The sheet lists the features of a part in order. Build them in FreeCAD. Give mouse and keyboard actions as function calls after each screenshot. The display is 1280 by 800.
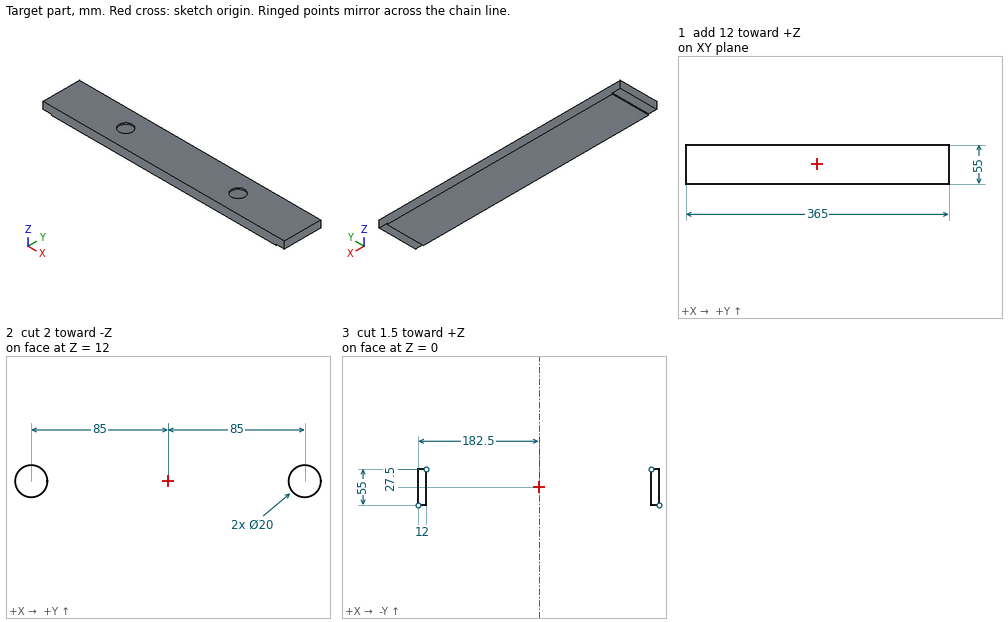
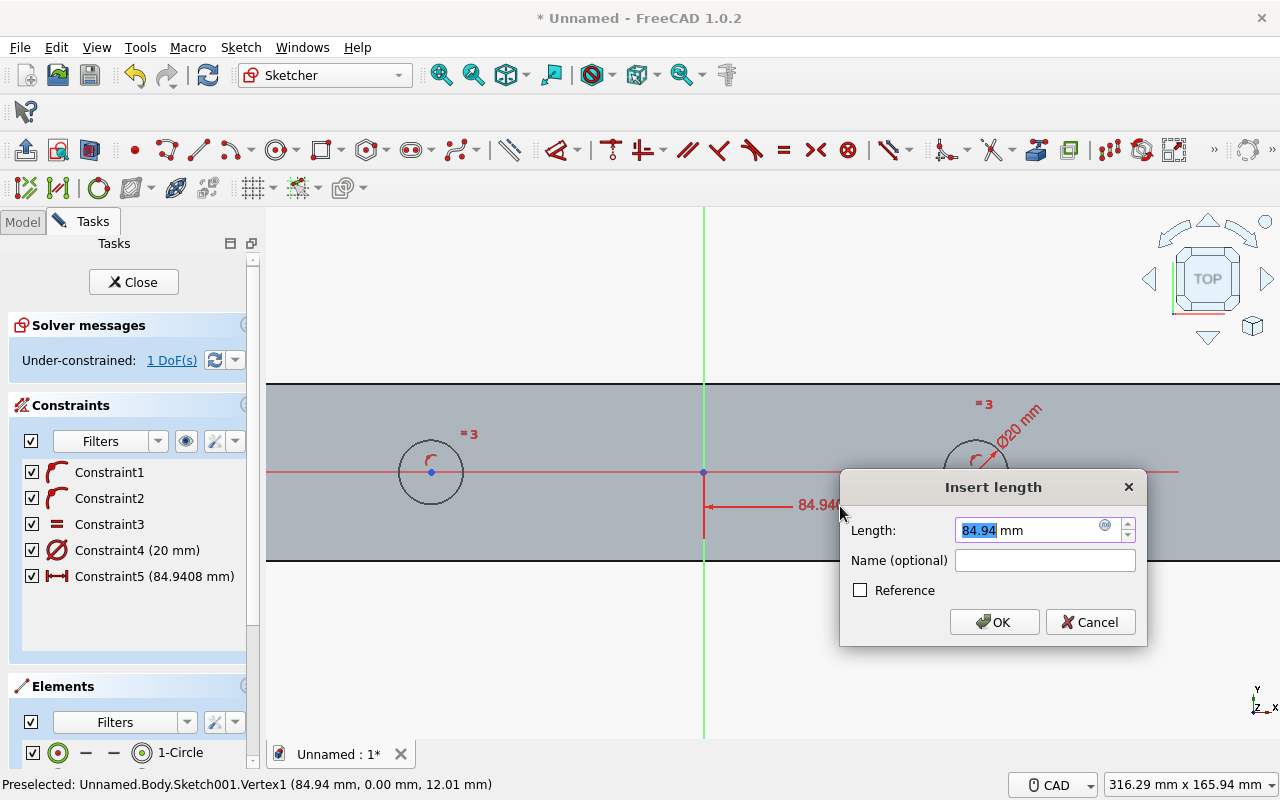
text(85)
key(Return)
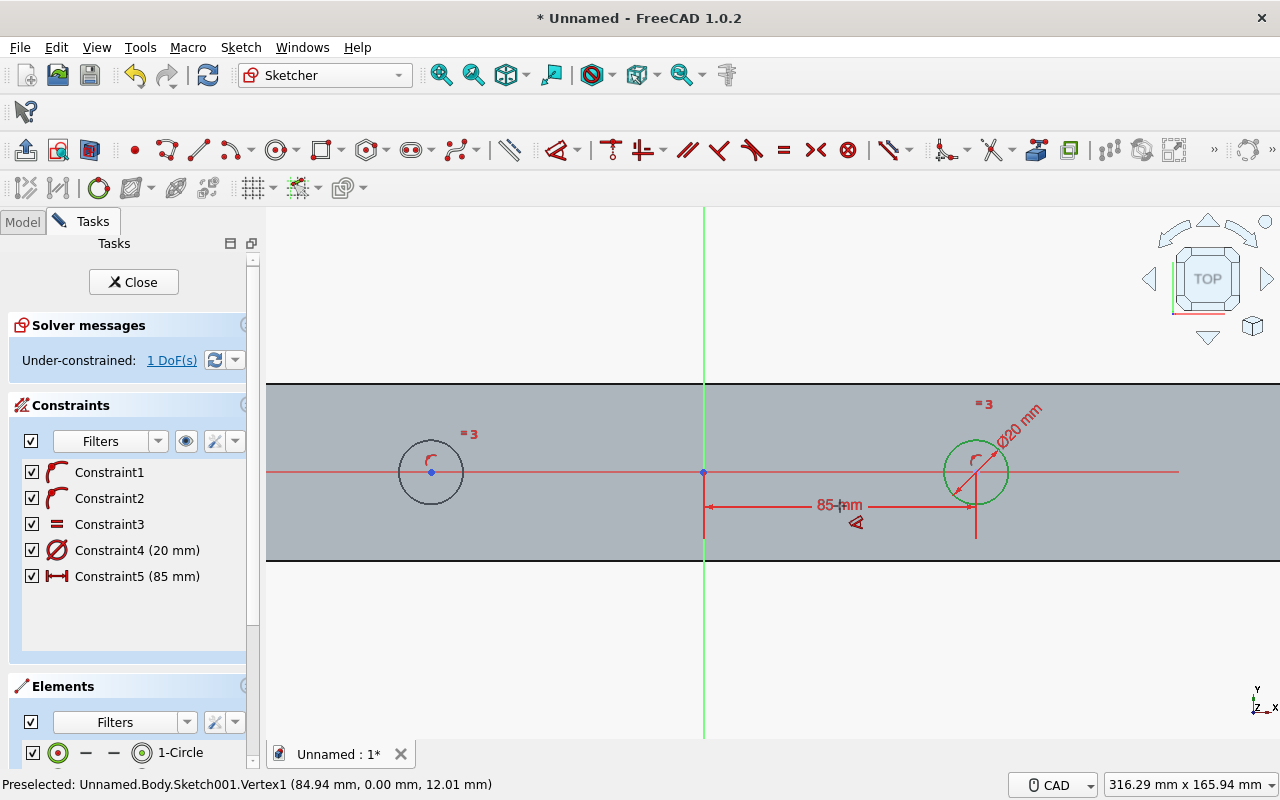
click(431, 472)
click(567, 506)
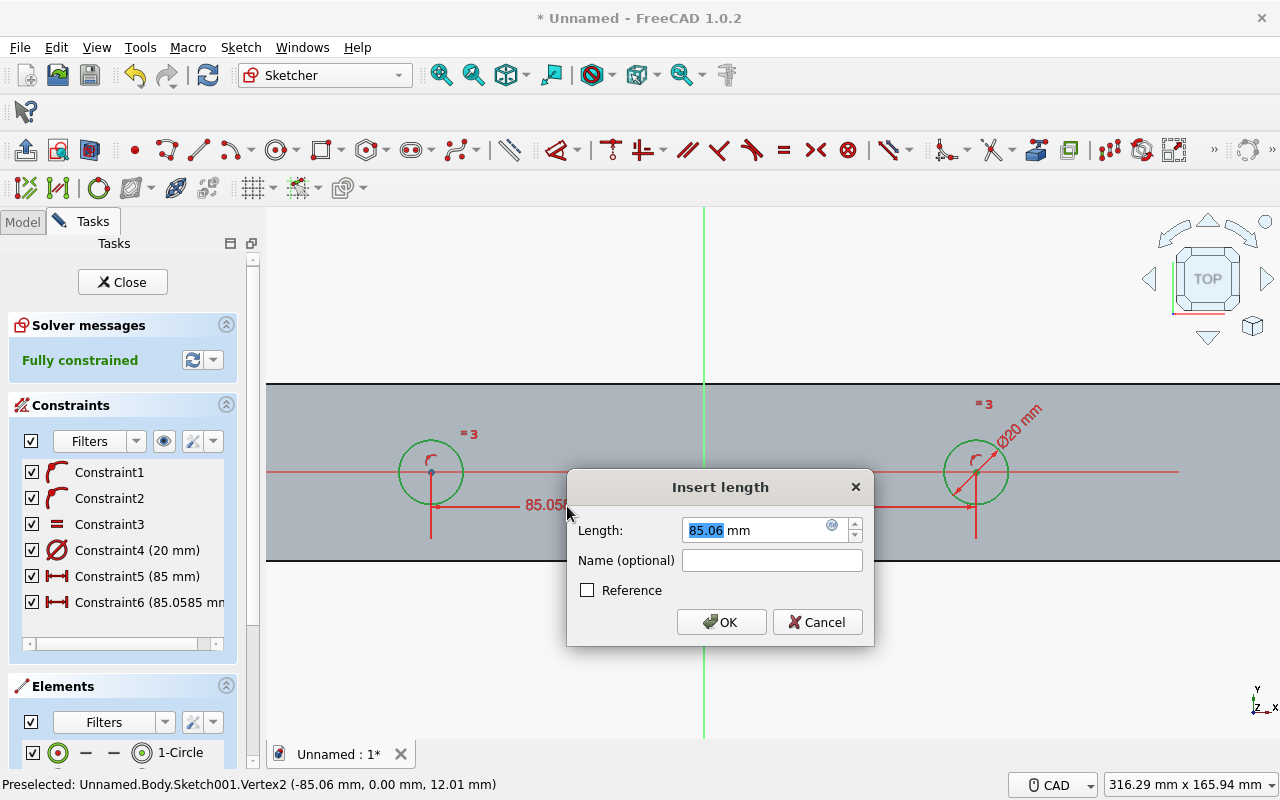
text(85)
key(Return)
key(Escape)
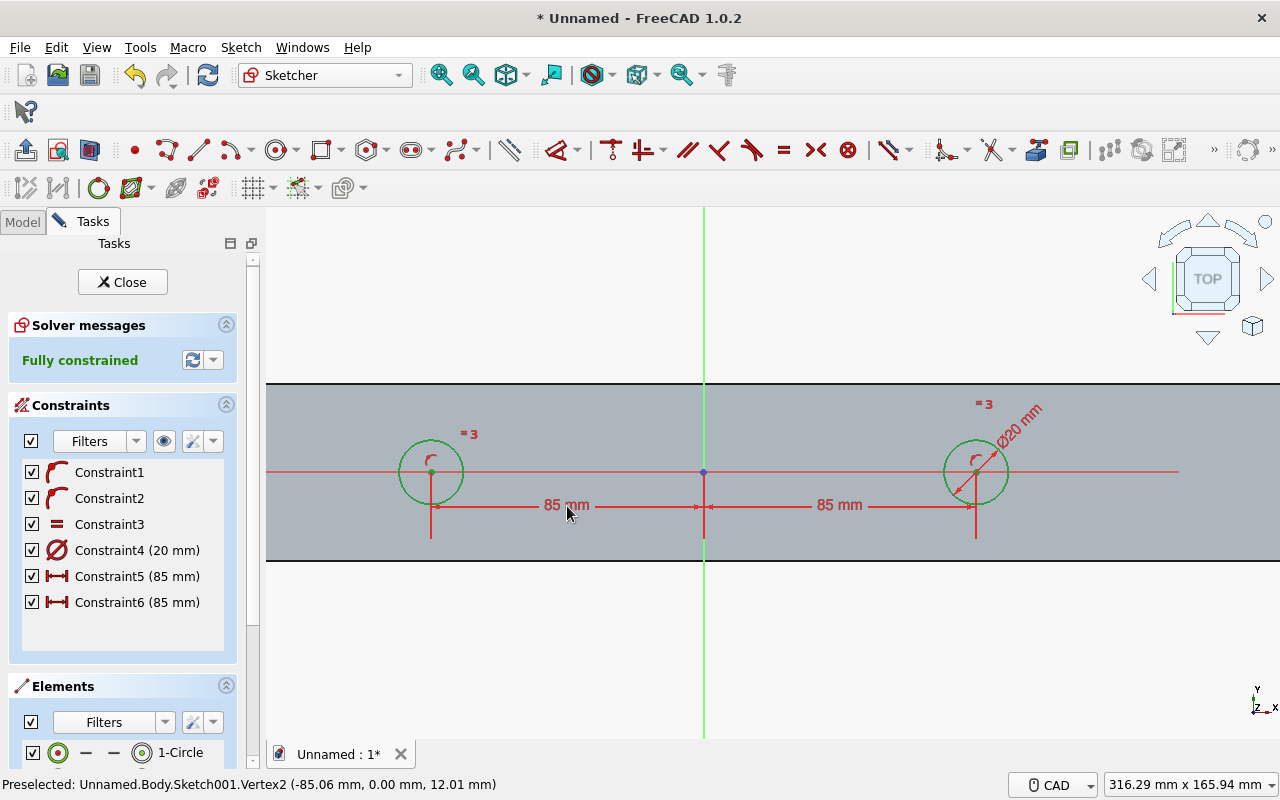
click(123, 282)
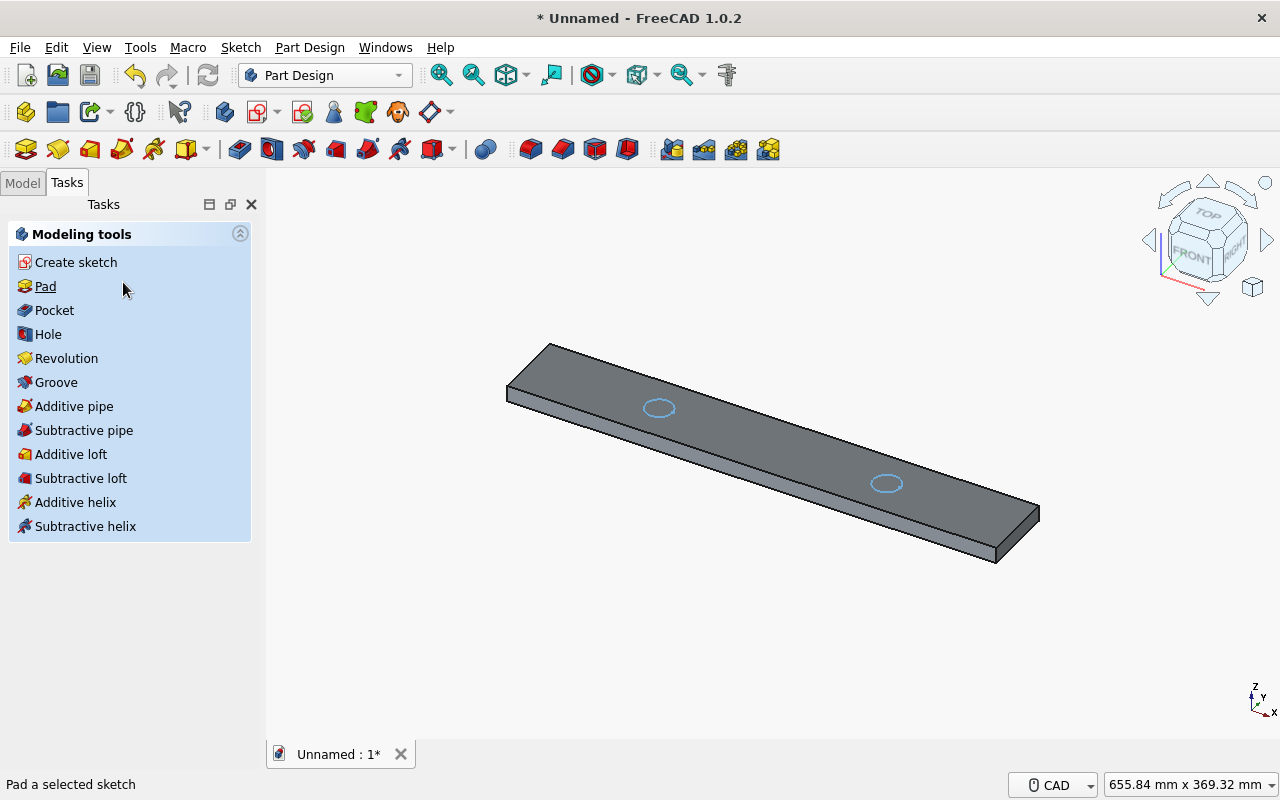
click(240, 150)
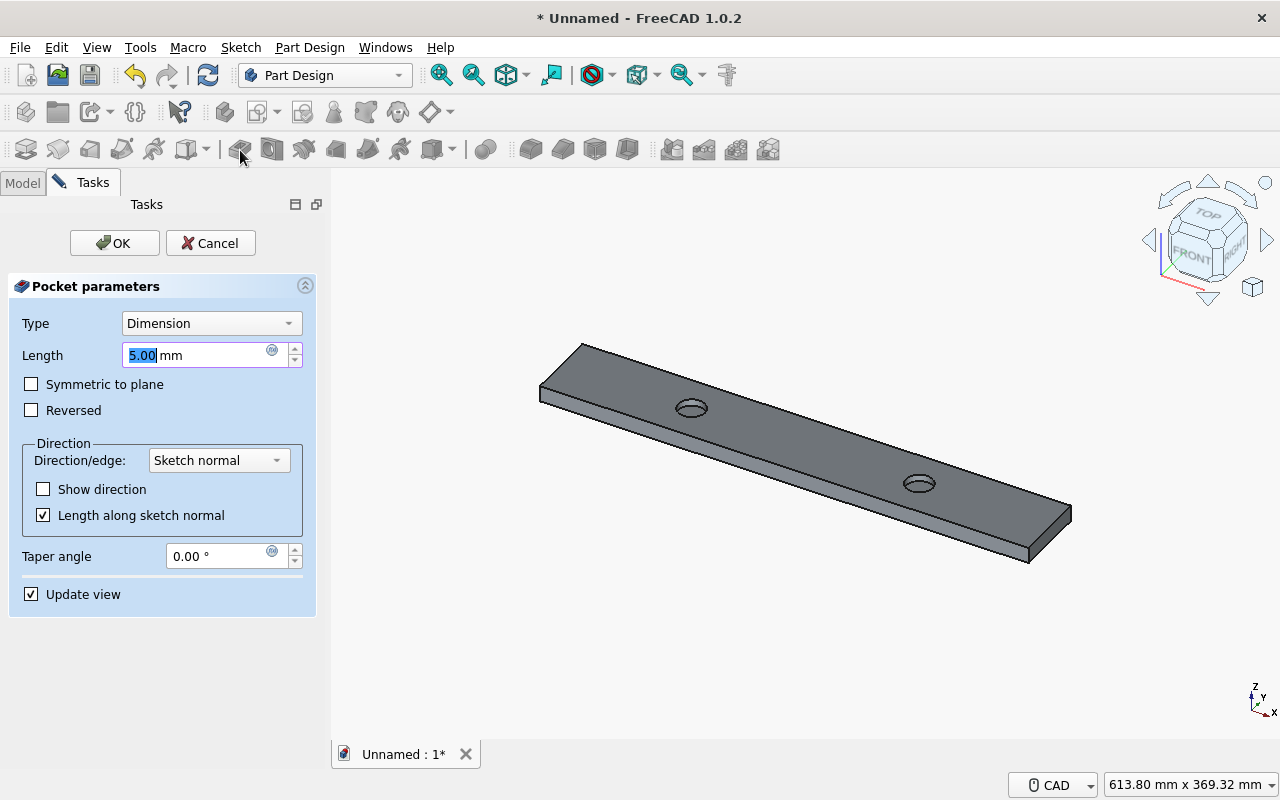
text(2)
key(Tab)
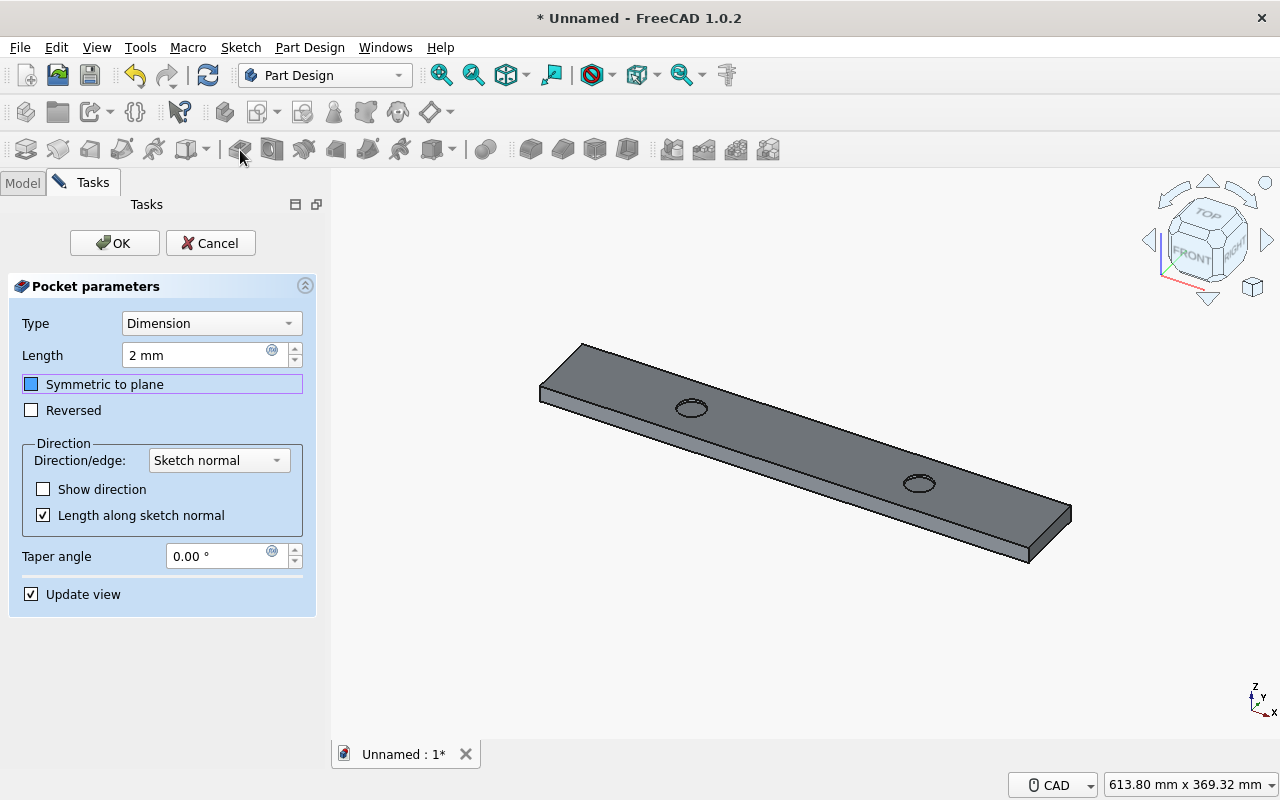
click(115, 243)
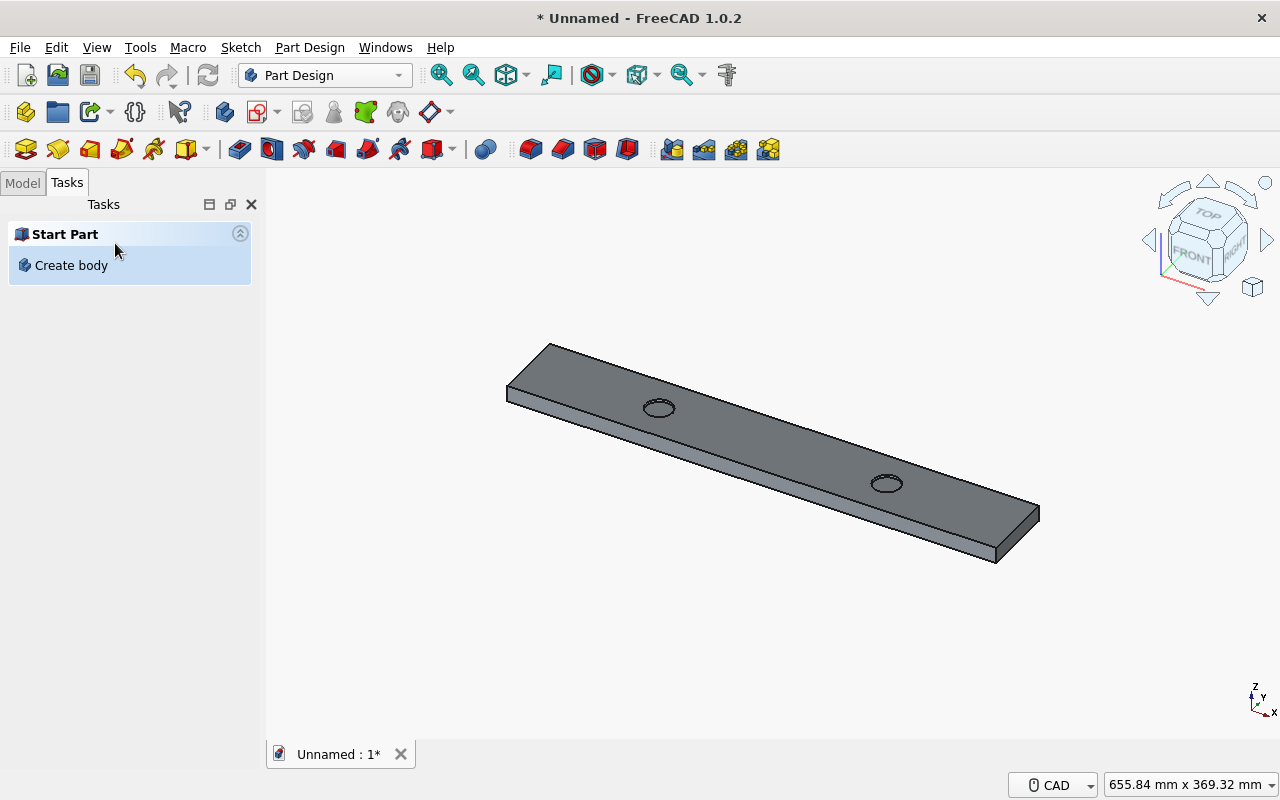
key(5)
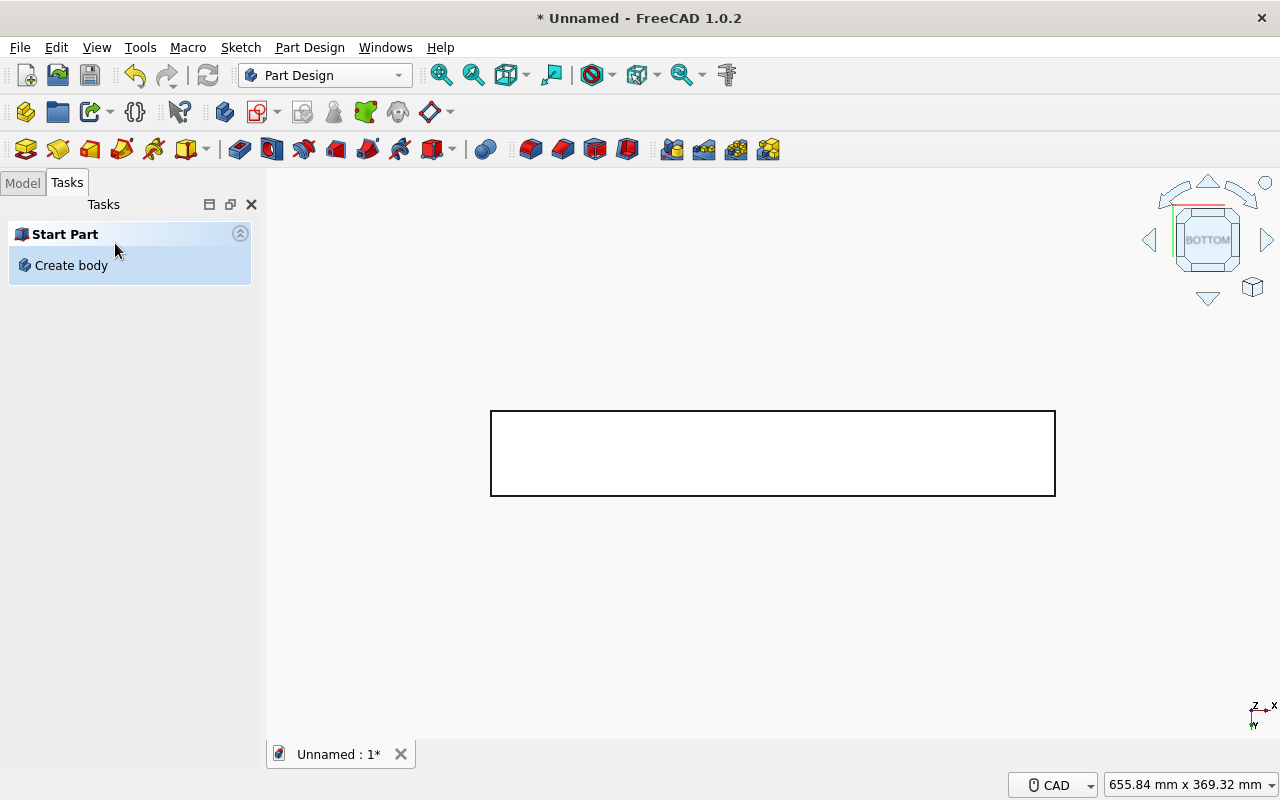
click(934, 452)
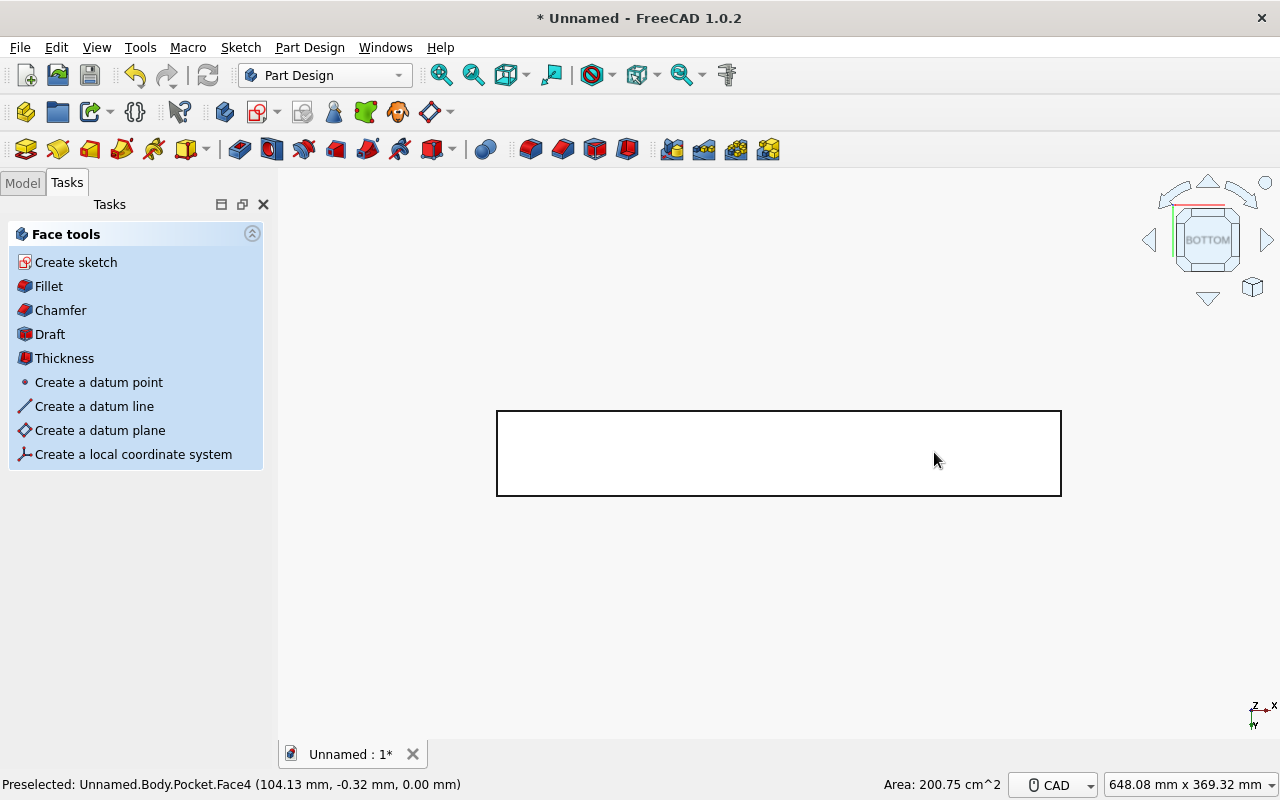
click(258, 112)